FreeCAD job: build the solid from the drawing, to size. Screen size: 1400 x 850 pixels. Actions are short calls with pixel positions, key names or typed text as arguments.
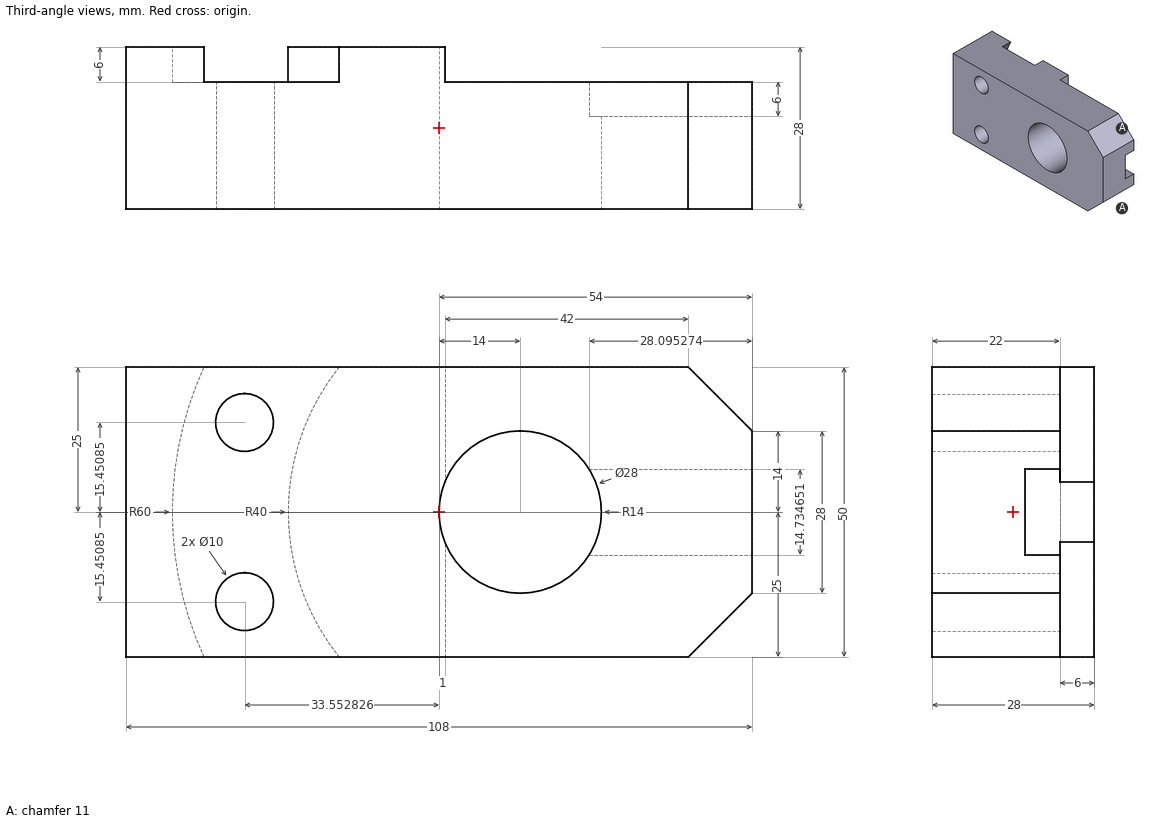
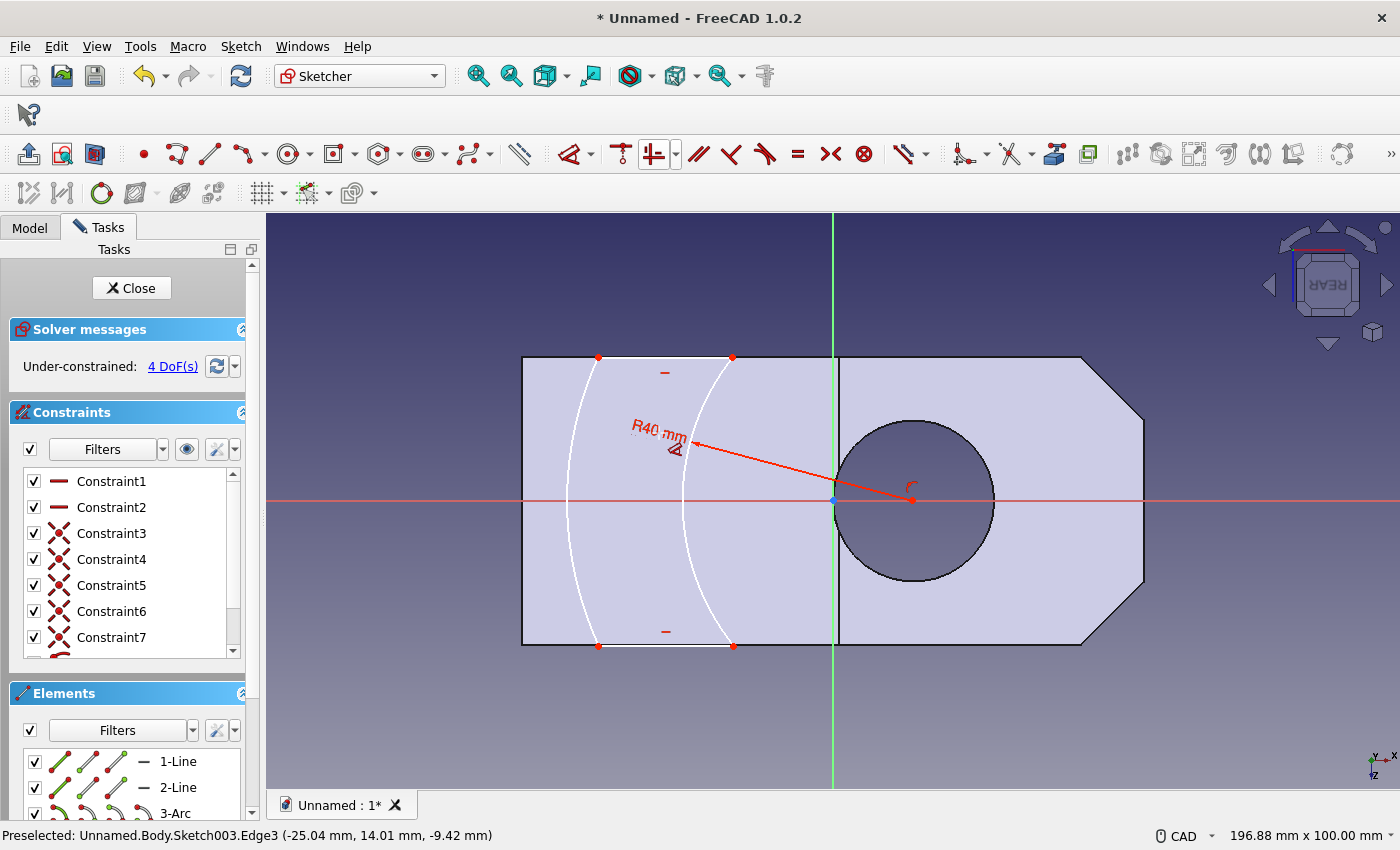
click(572, 443)
click(540, 438)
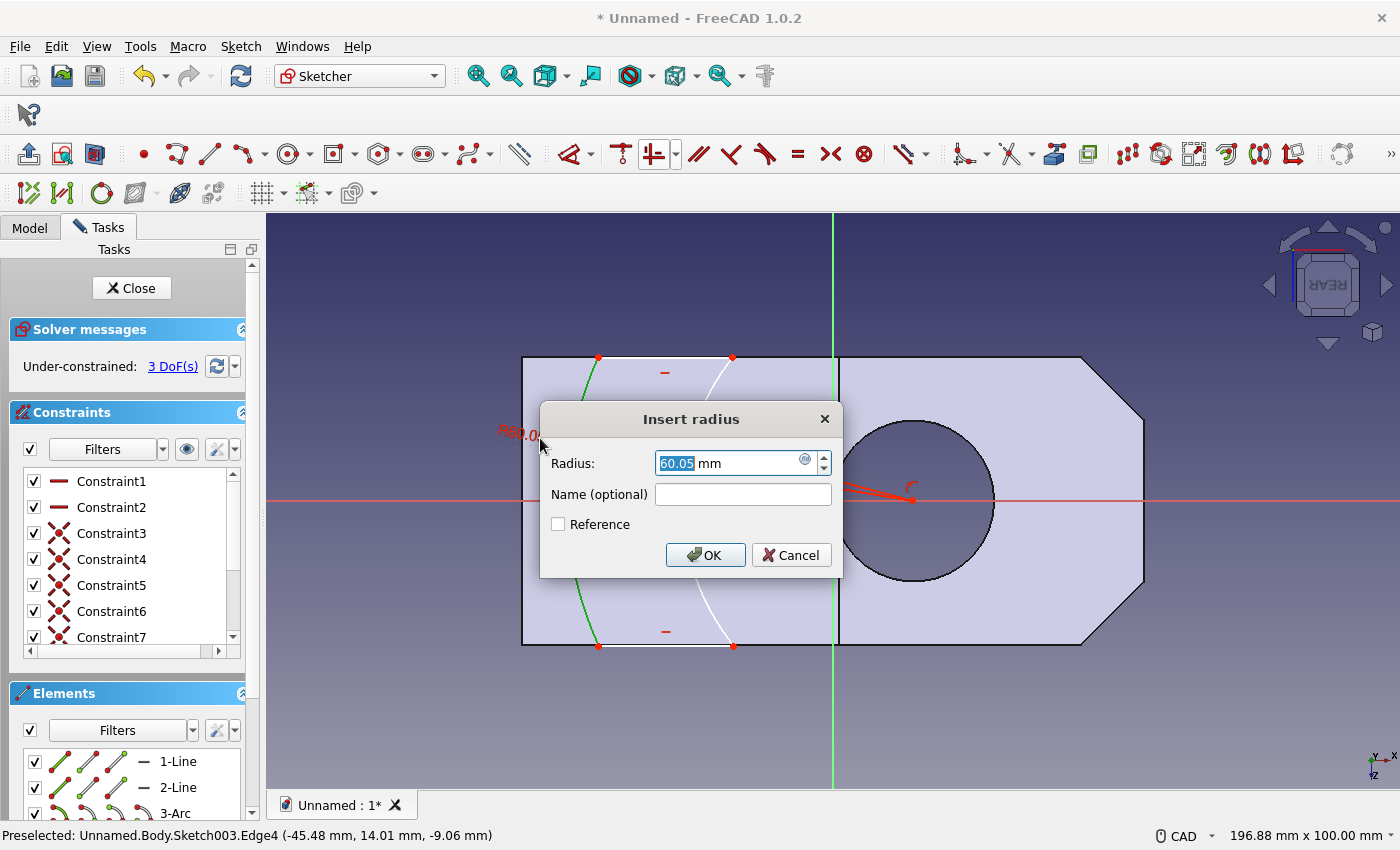
text(60)
key(Return)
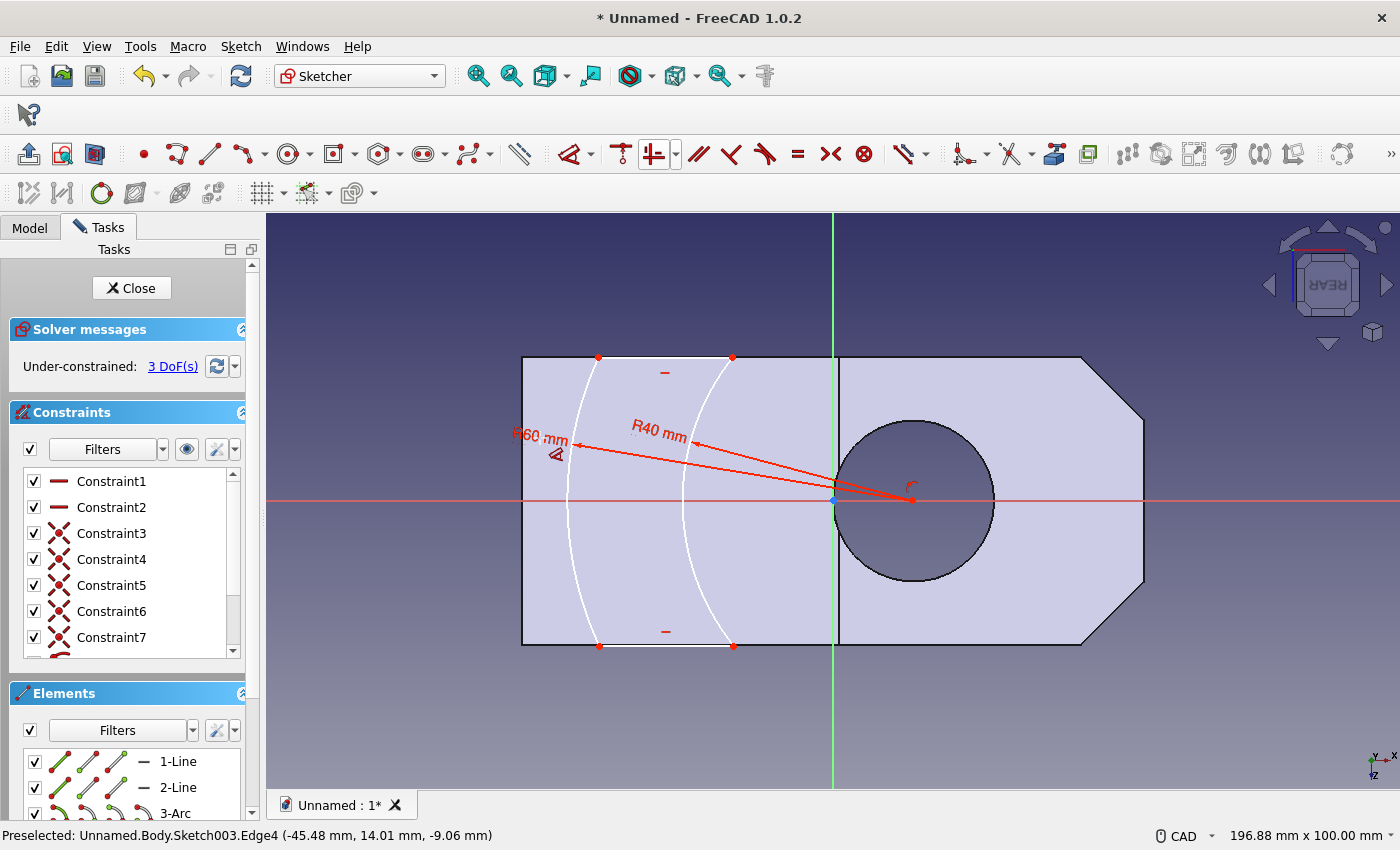
click(599, 646)
click(867, 574)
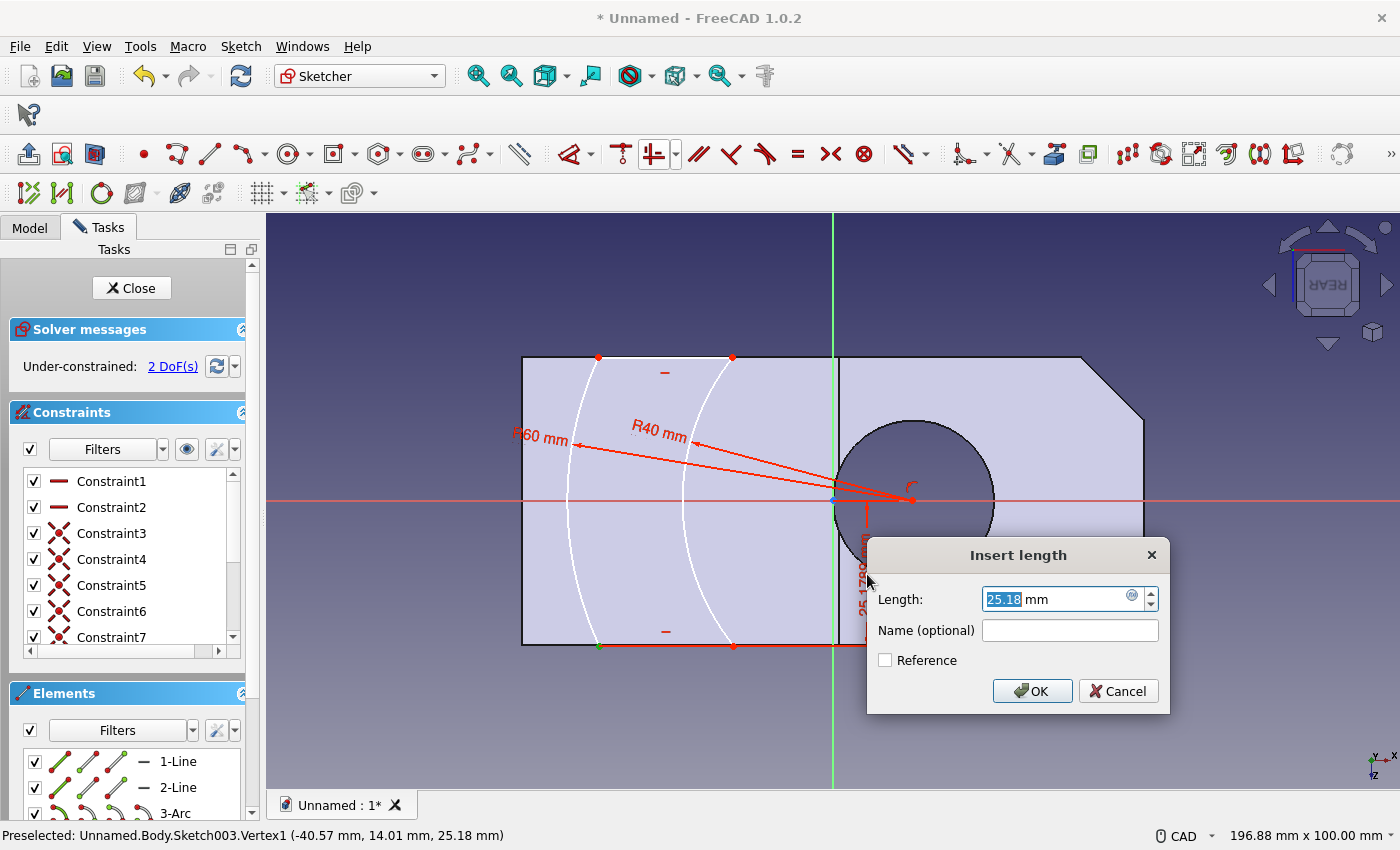
text(25)
key(Return)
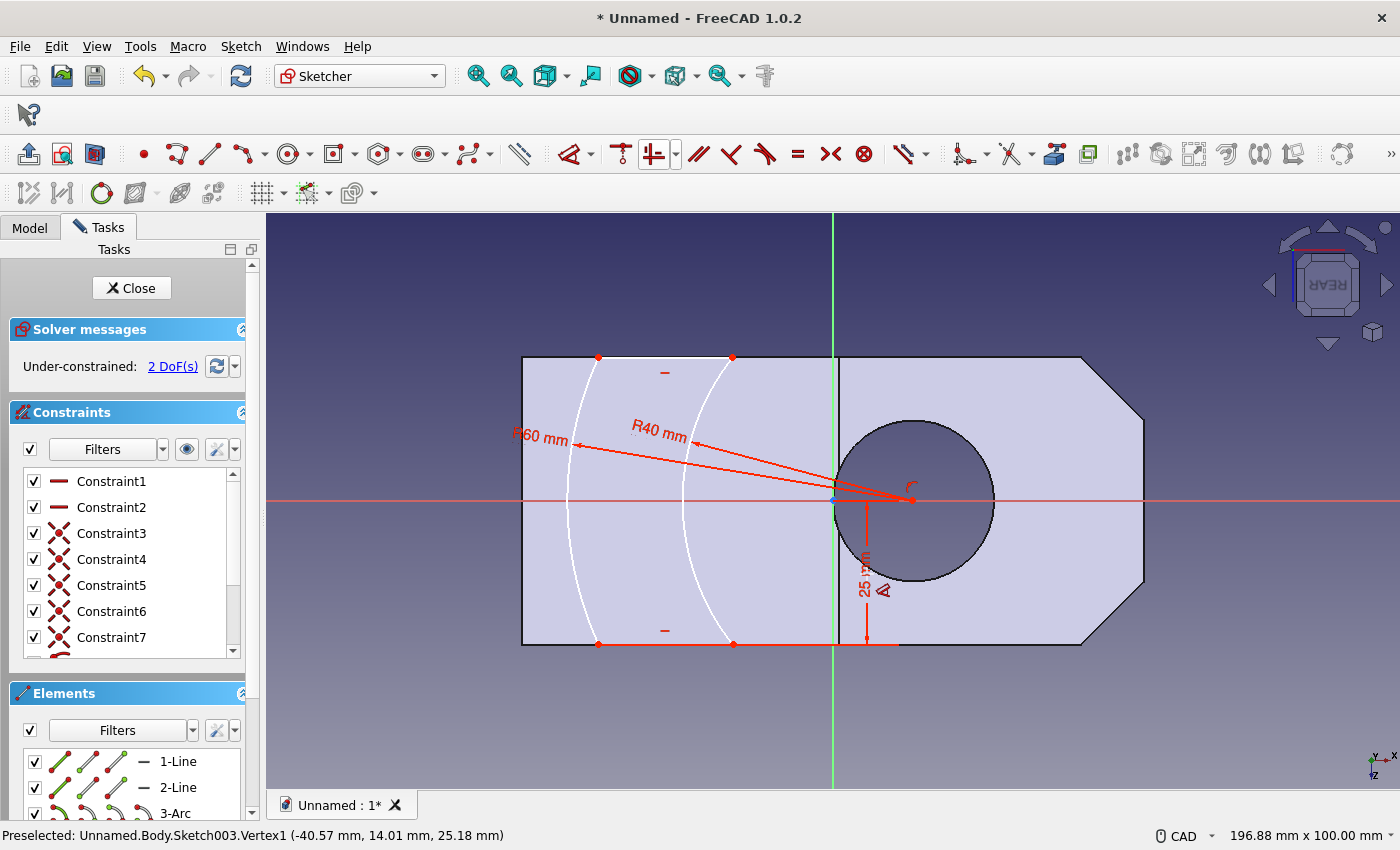
click(732, 358)
click(867, 429)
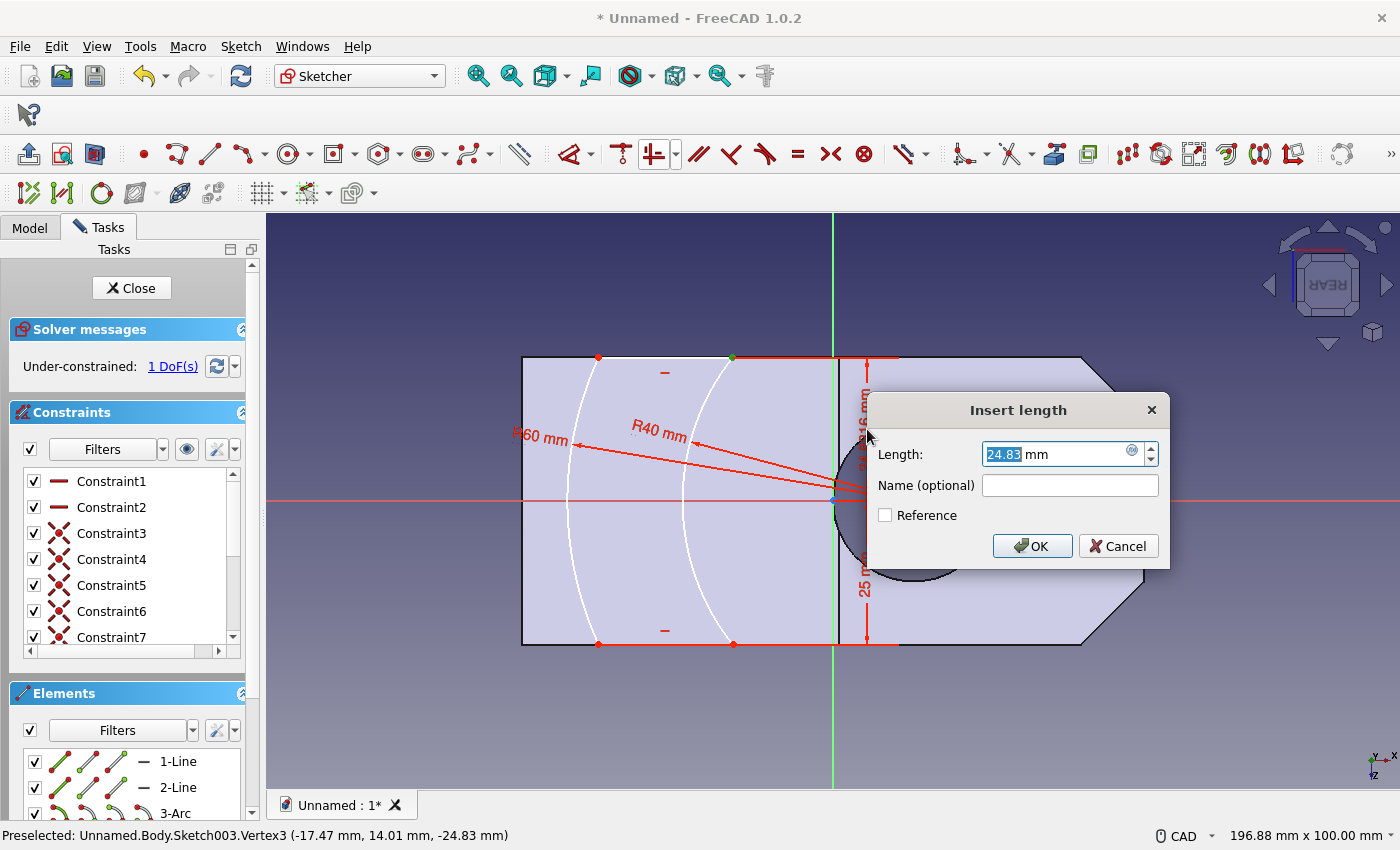
text(25)
key(Return)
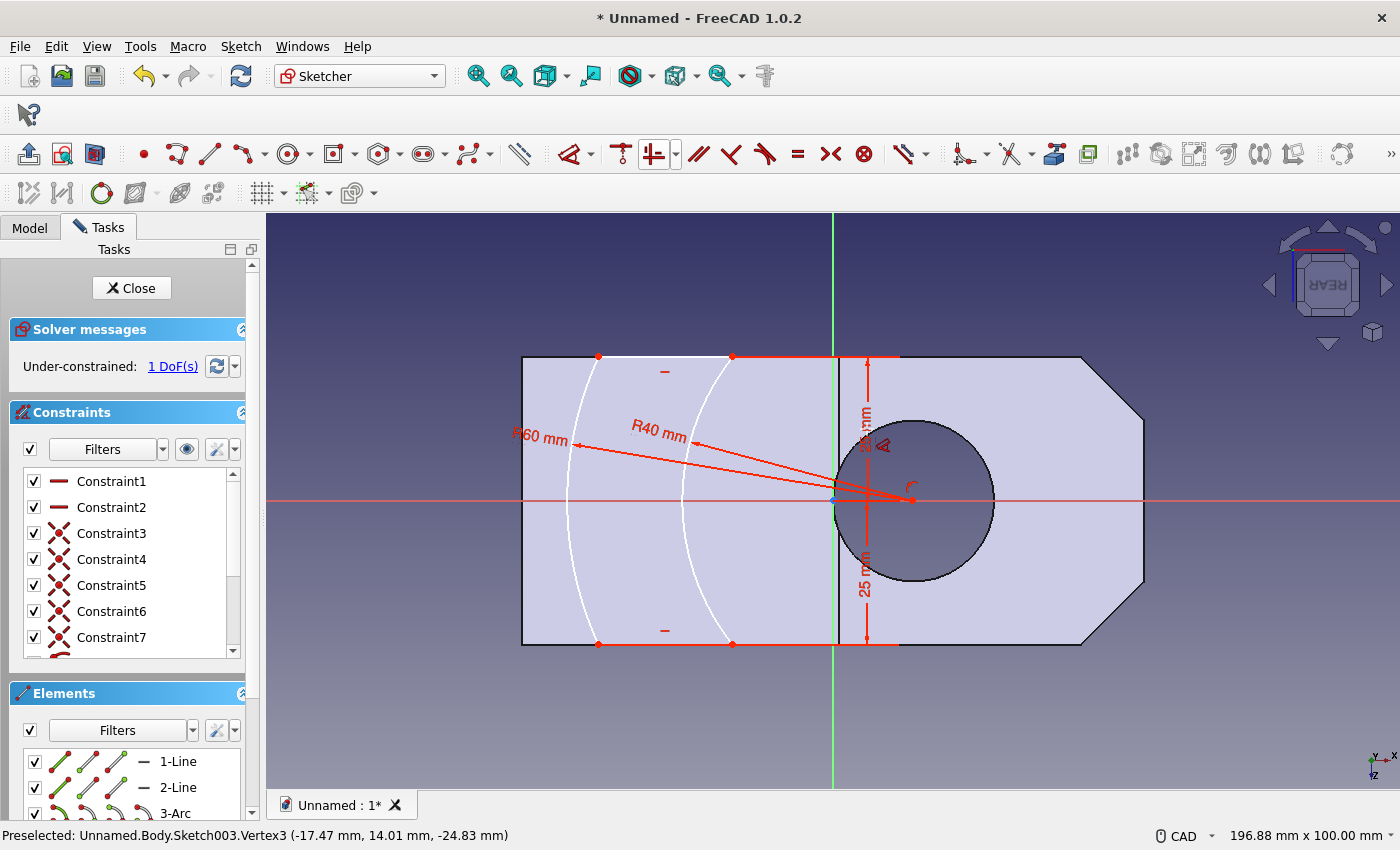
click(913, 501)
click(873, 535)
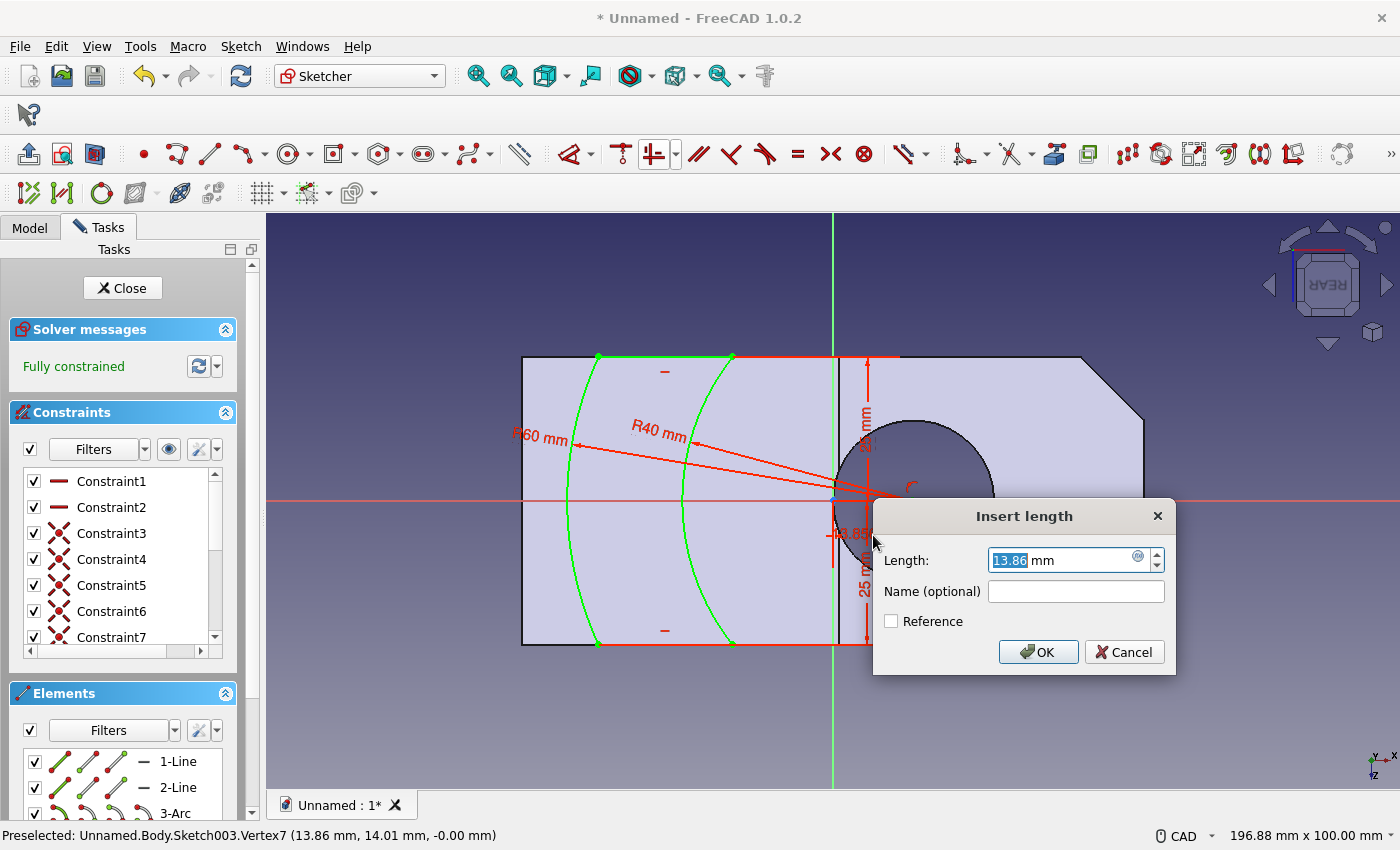
text(14)
key(Return)
key(Escape)